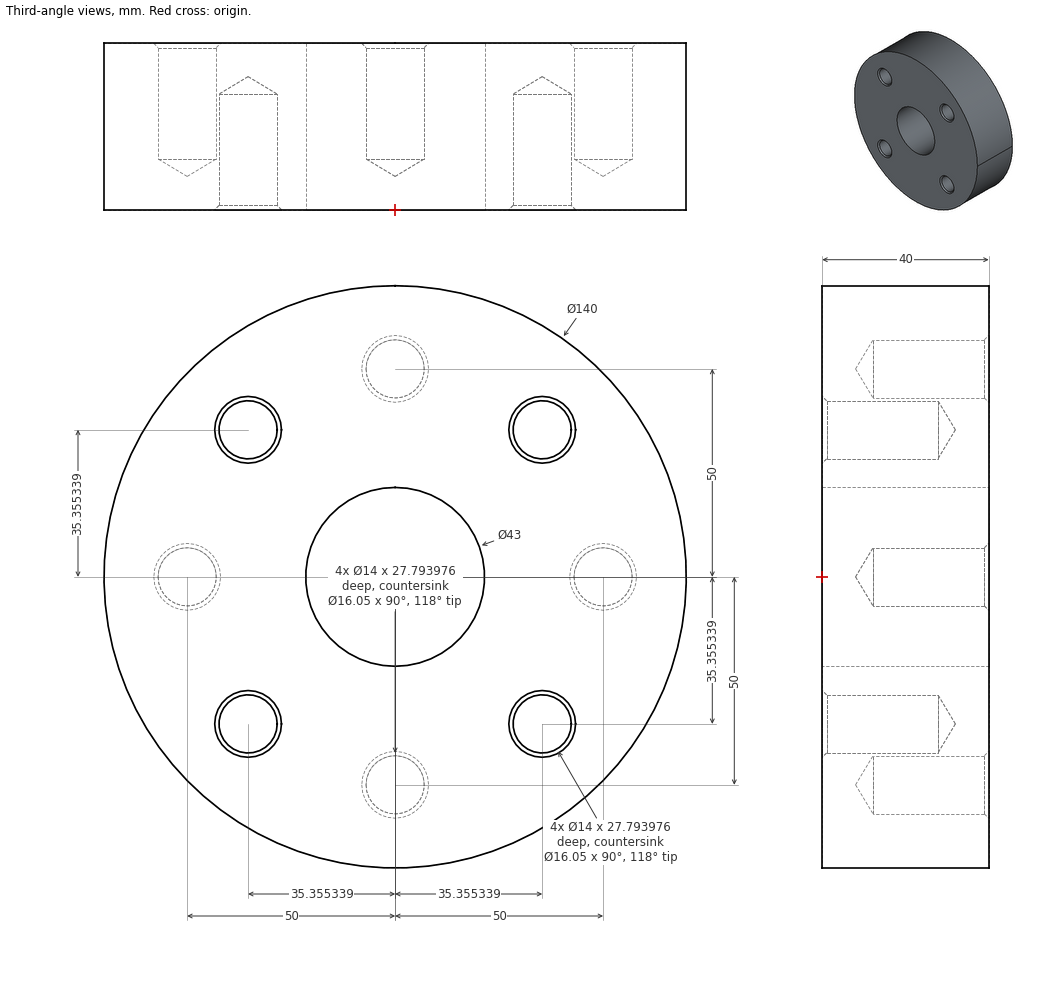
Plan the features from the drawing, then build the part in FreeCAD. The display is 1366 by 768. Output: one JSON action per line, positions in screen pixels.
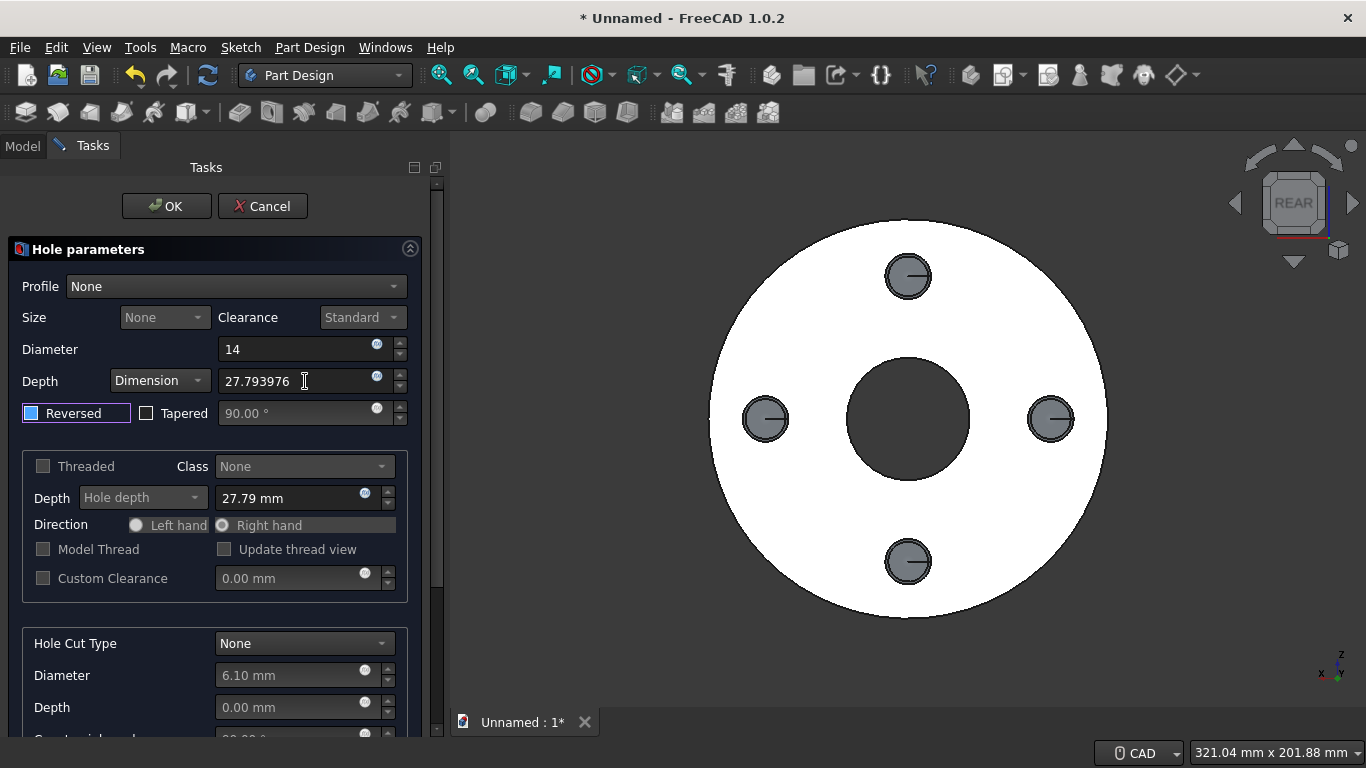
{"action": "left_click", "coordinate": [306, 644]}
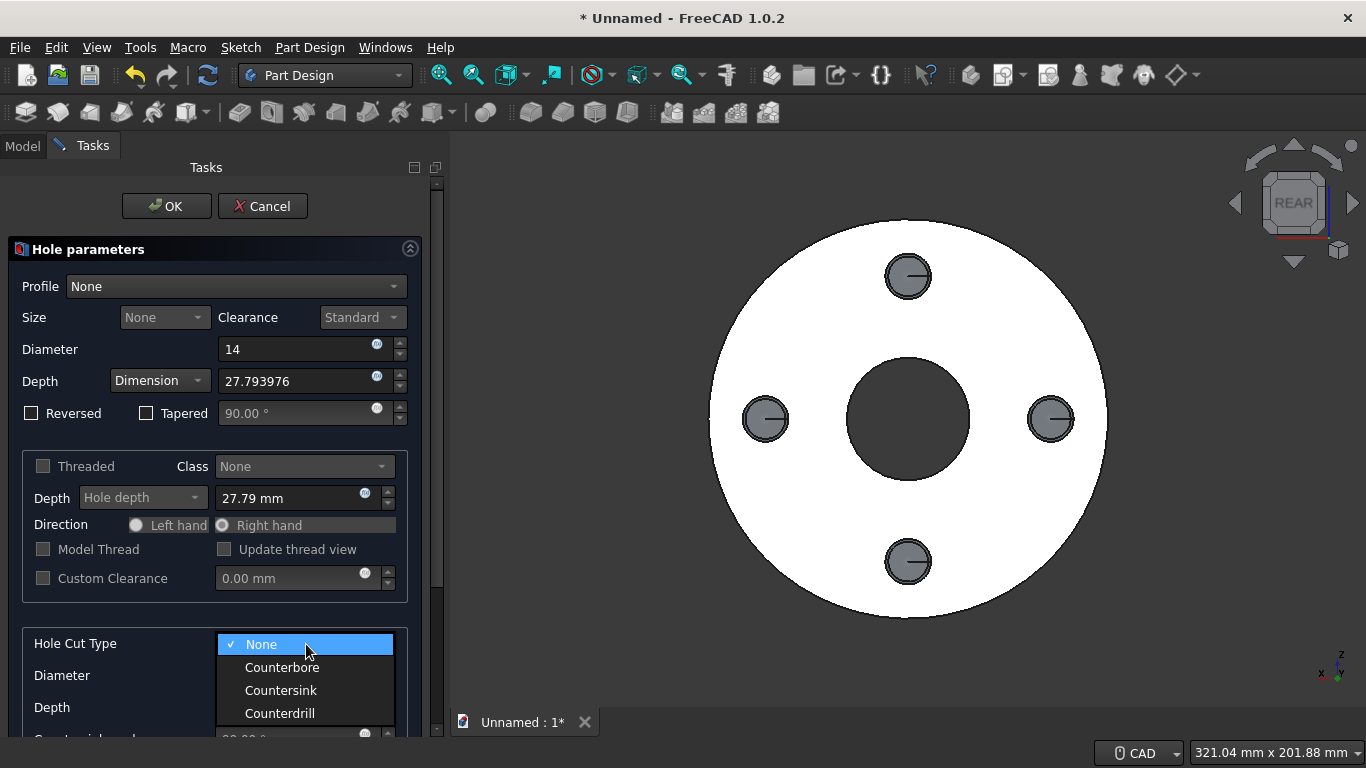
{"action": "left_click", "coordinate": [304, 690]}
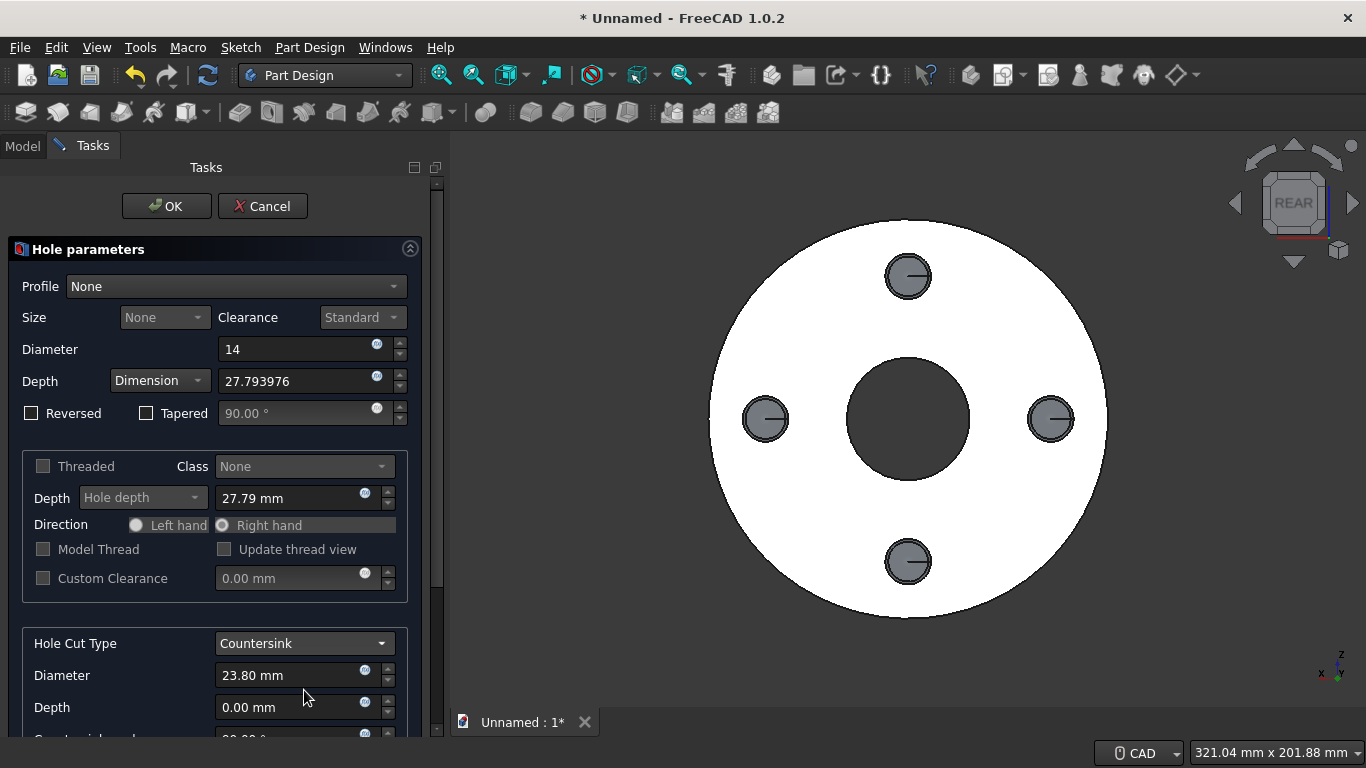
{"action": "triple_click", "coordinate": [298, 675]}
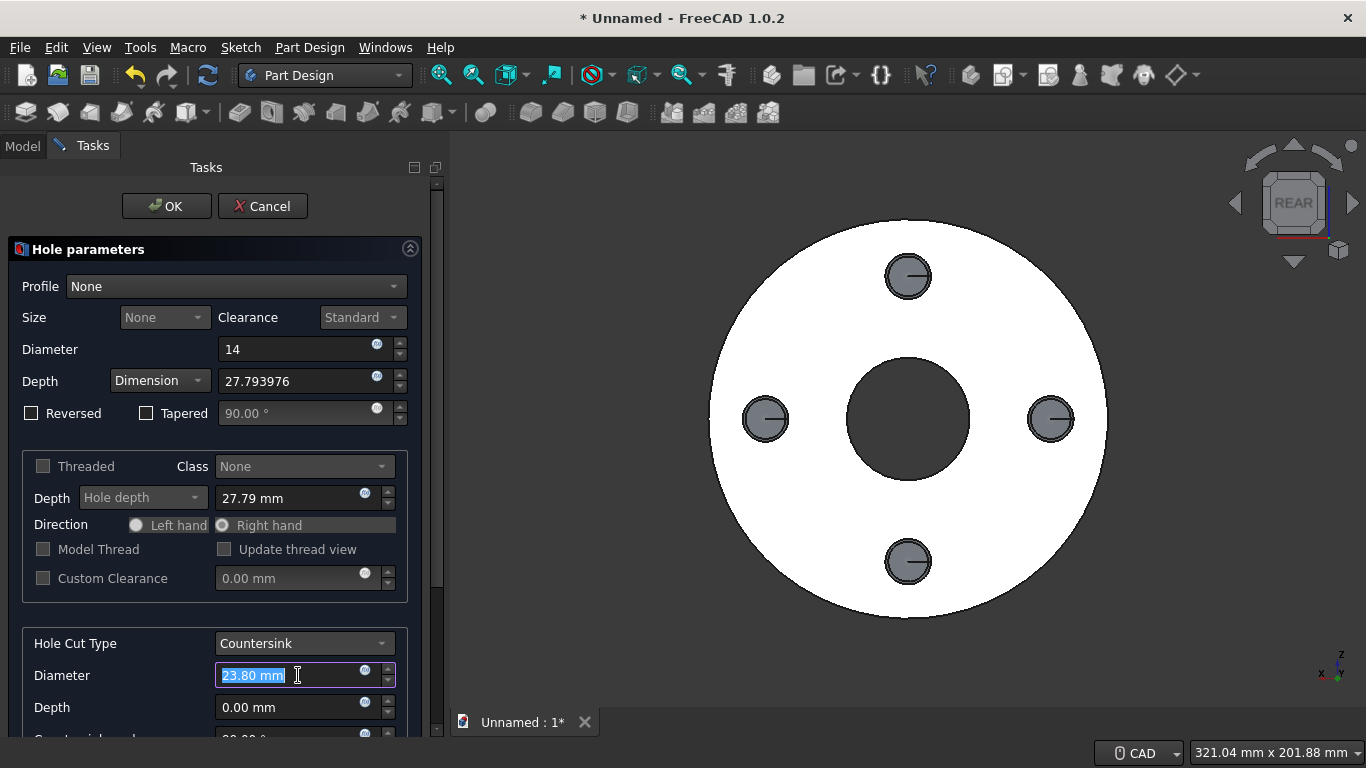
{"action": "type", "text": "16.05"}
{"action": "key", "text": "Tab"}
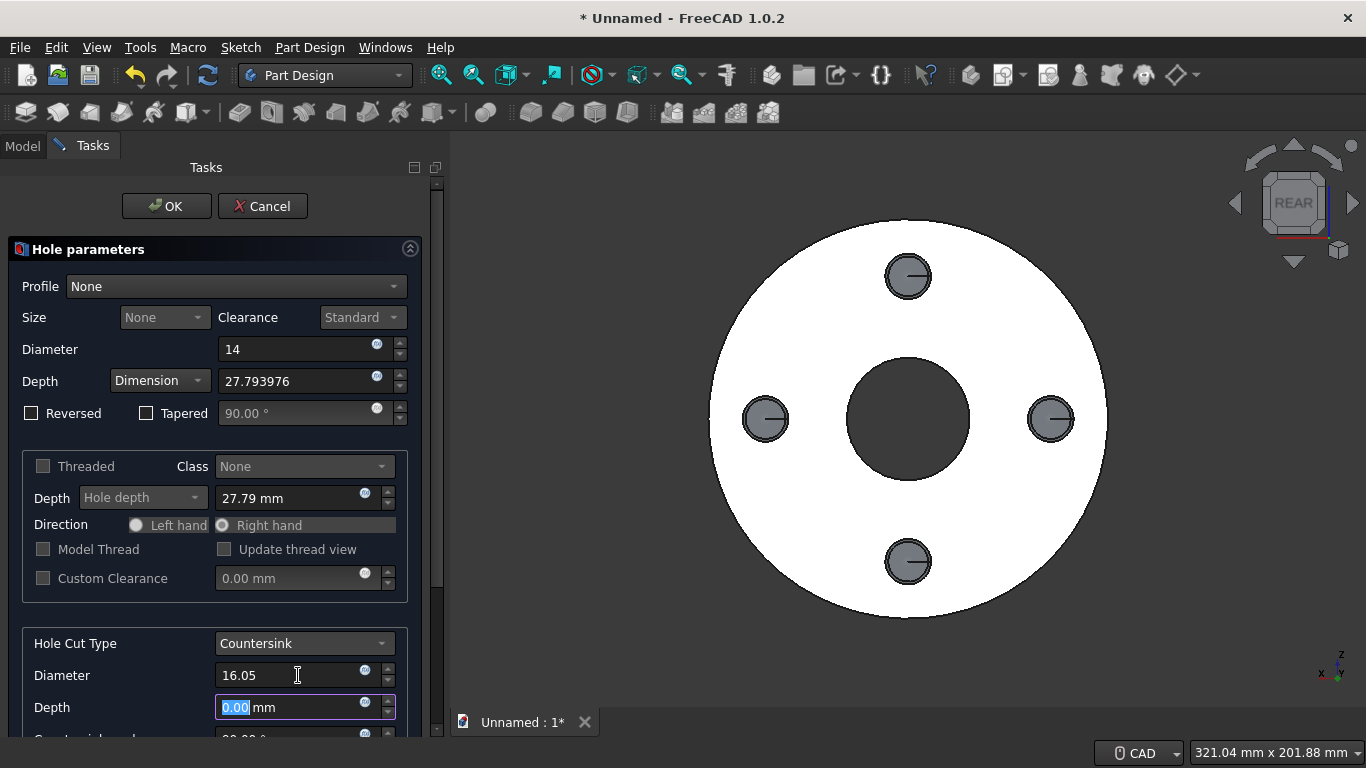
{"action": "left_click", "coordinate": [167, 206]}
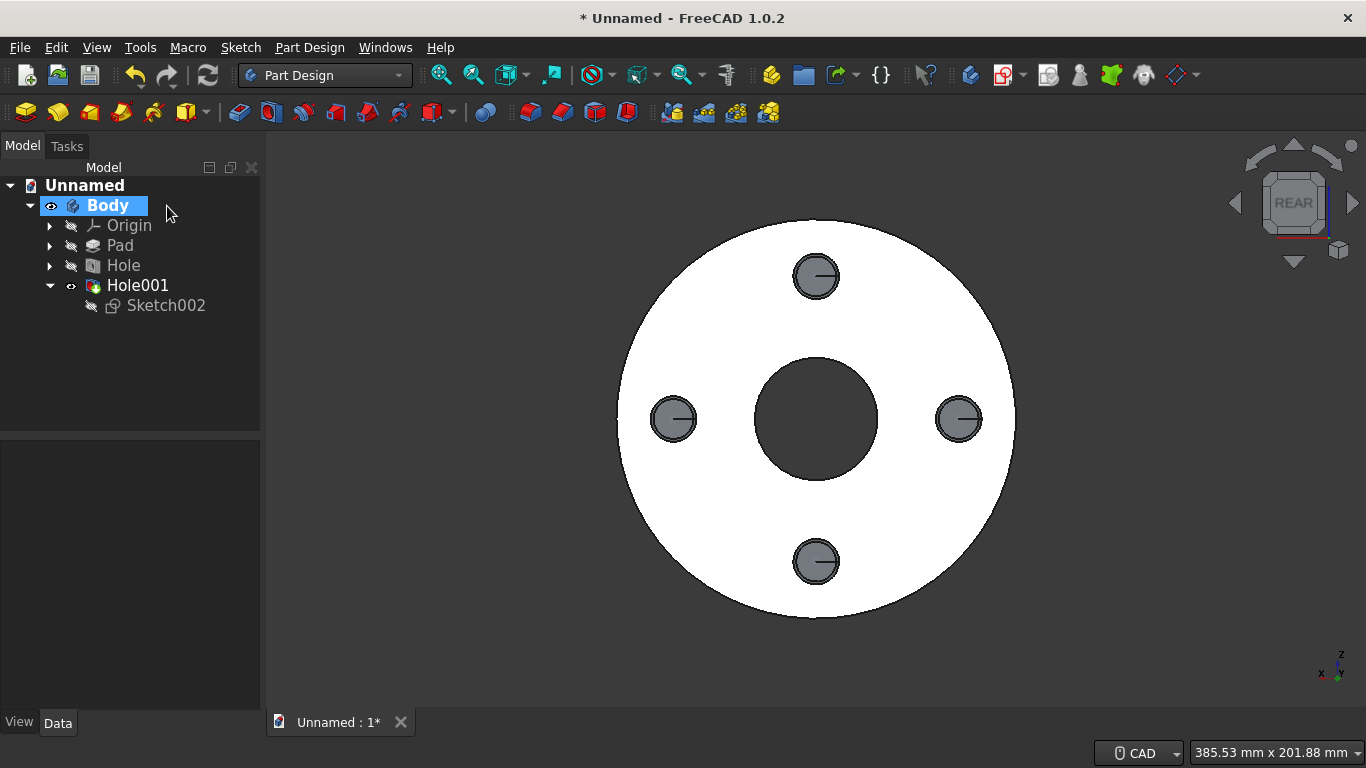
{"action": "key", "text": "0"}